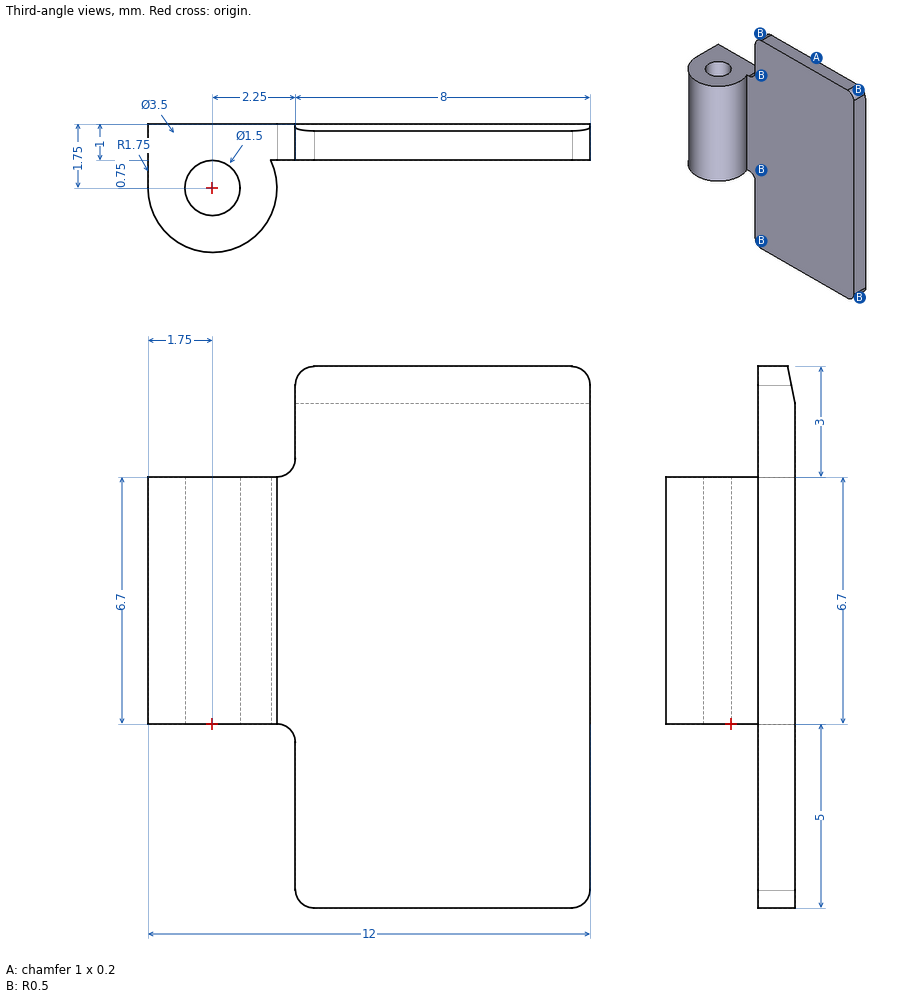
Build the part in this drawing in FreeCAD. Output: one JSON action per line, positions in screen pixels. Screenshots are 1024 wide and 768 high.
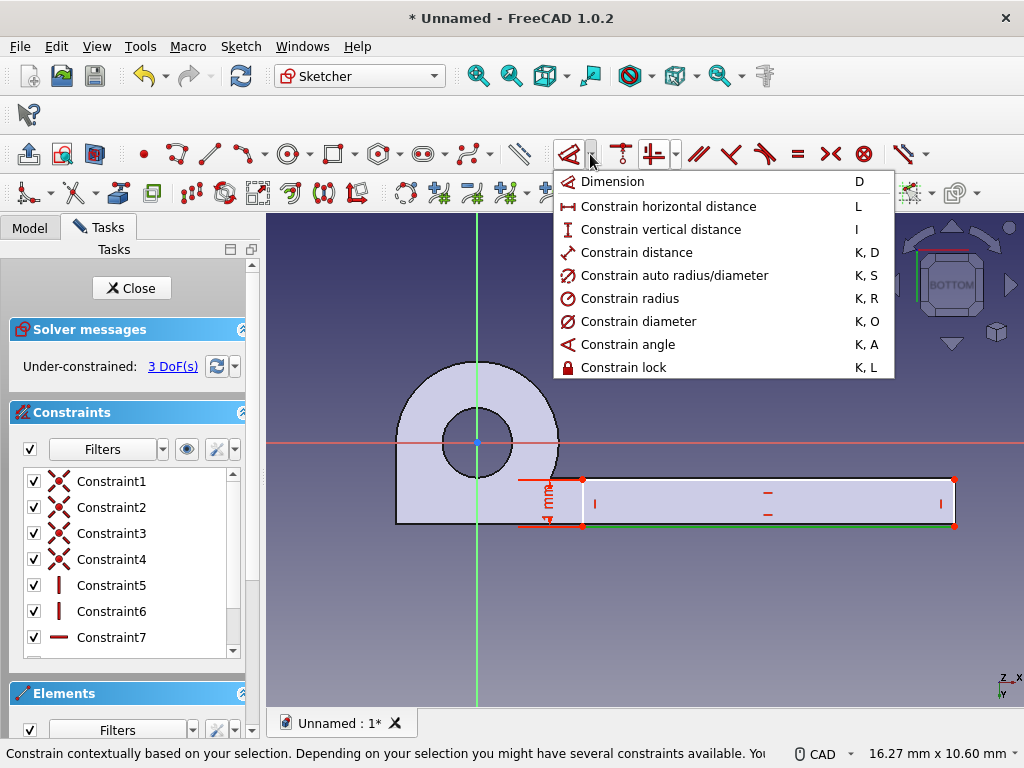
{"action": "left_click", "coordinate": [724, 206]}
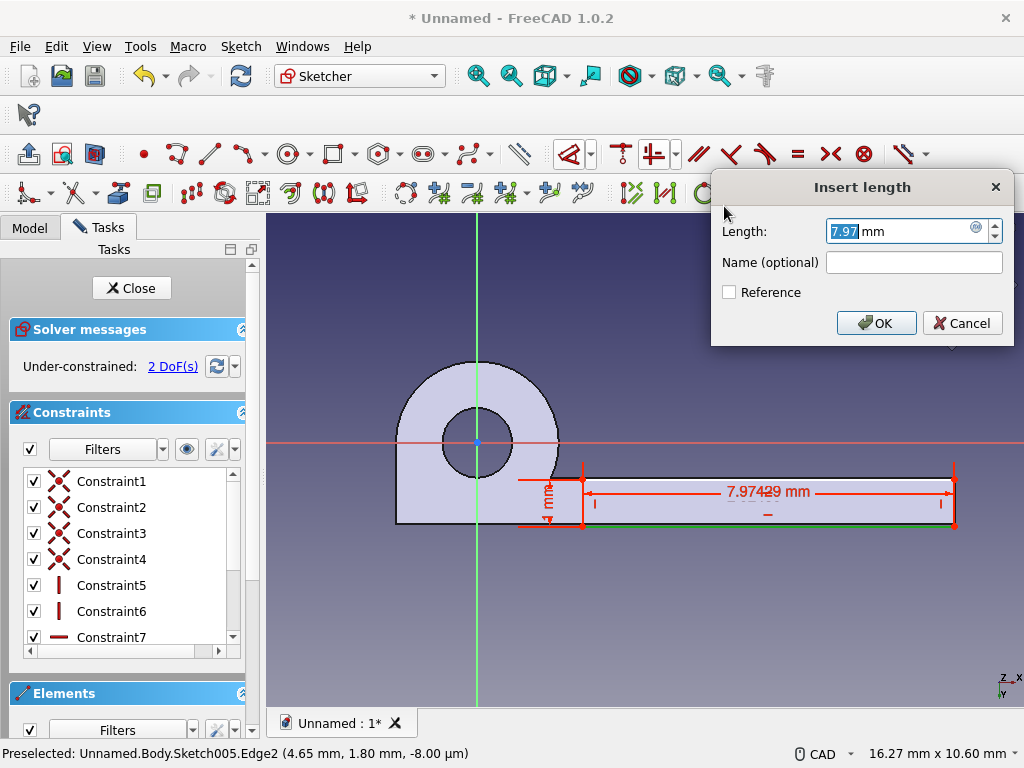
{"action": "type", "text": "8"}
{"action": "key", "text": "Return"}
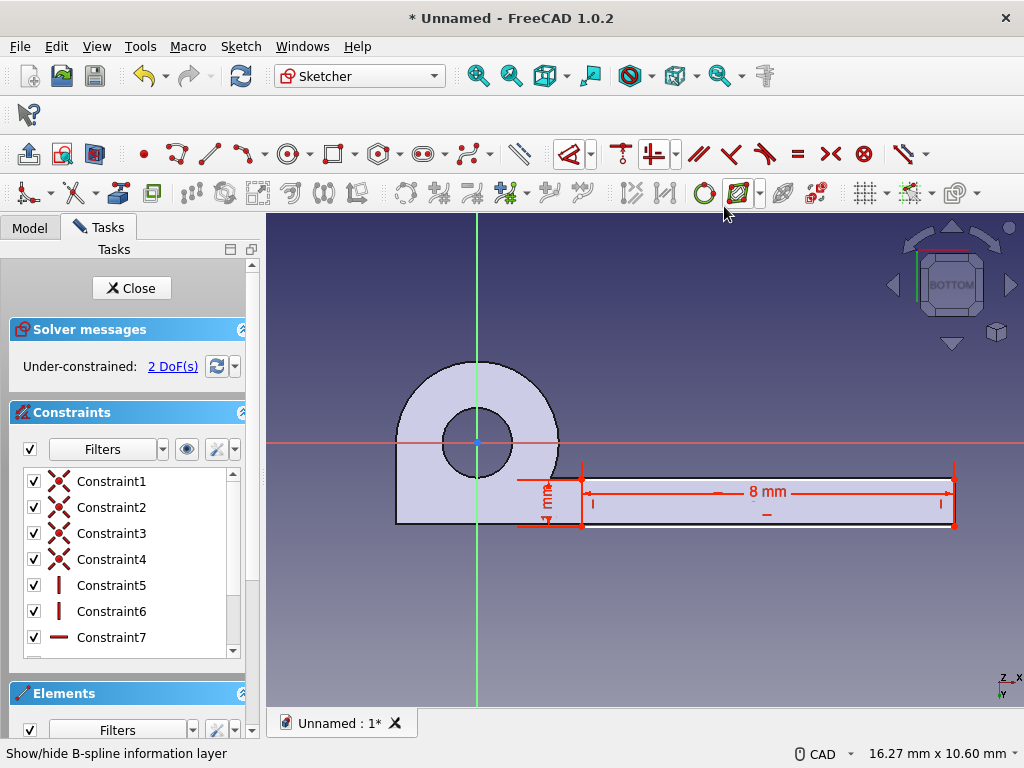
{"action": "left_click", "coordinate": [582, 480]}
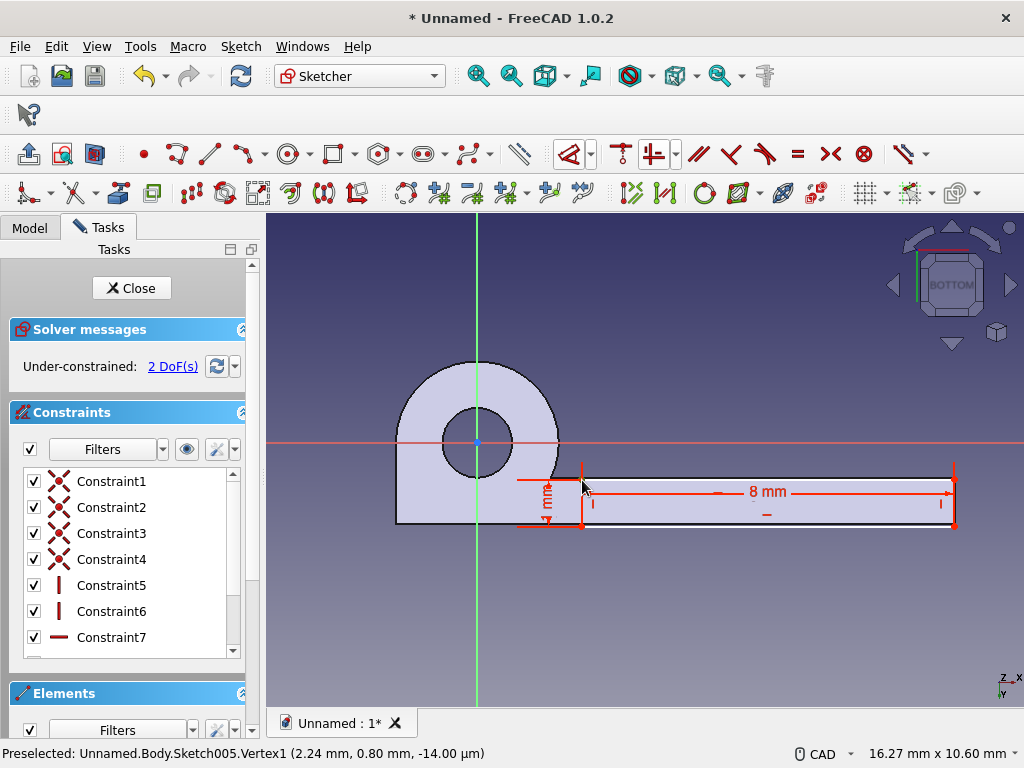
{"action": "key", "text": "l"}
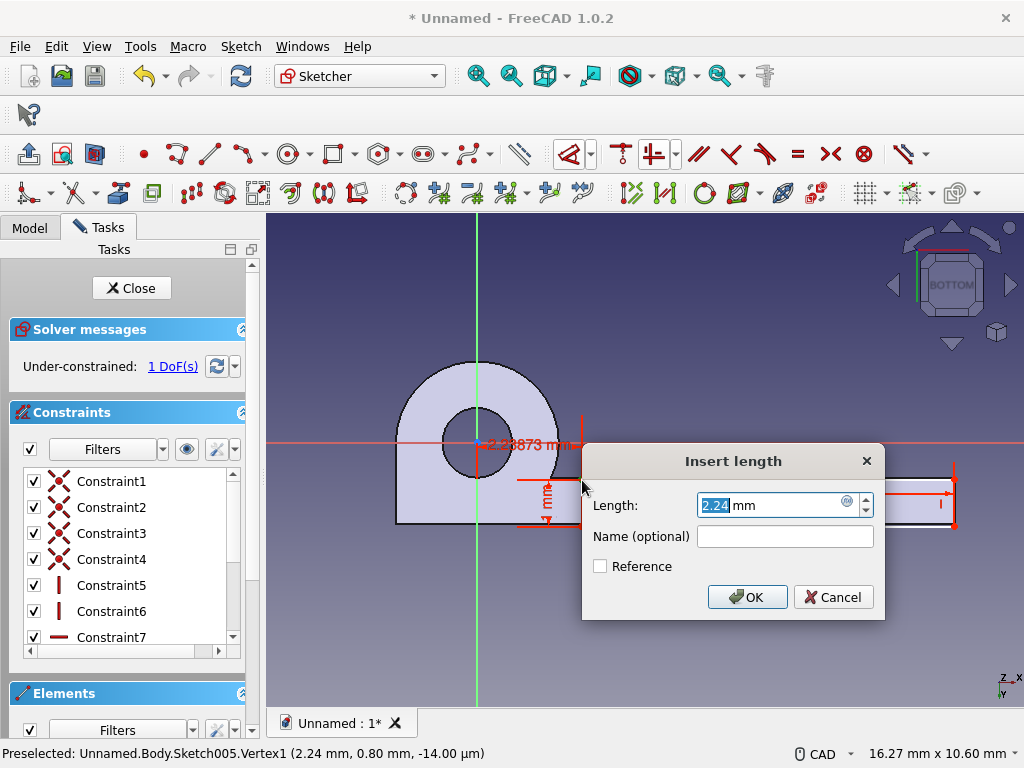
{"action": "type", "text": "2.25"}
{"action": "key", "text": "Return"}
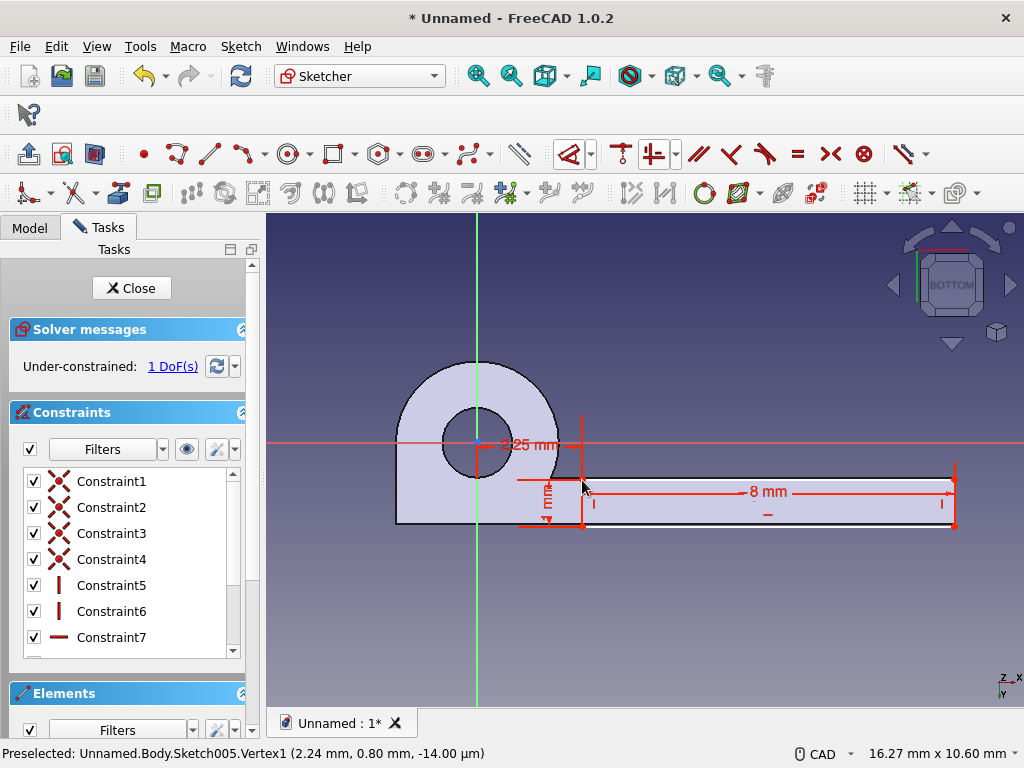
{"action": "left_click", "coordinate": [582, 480]}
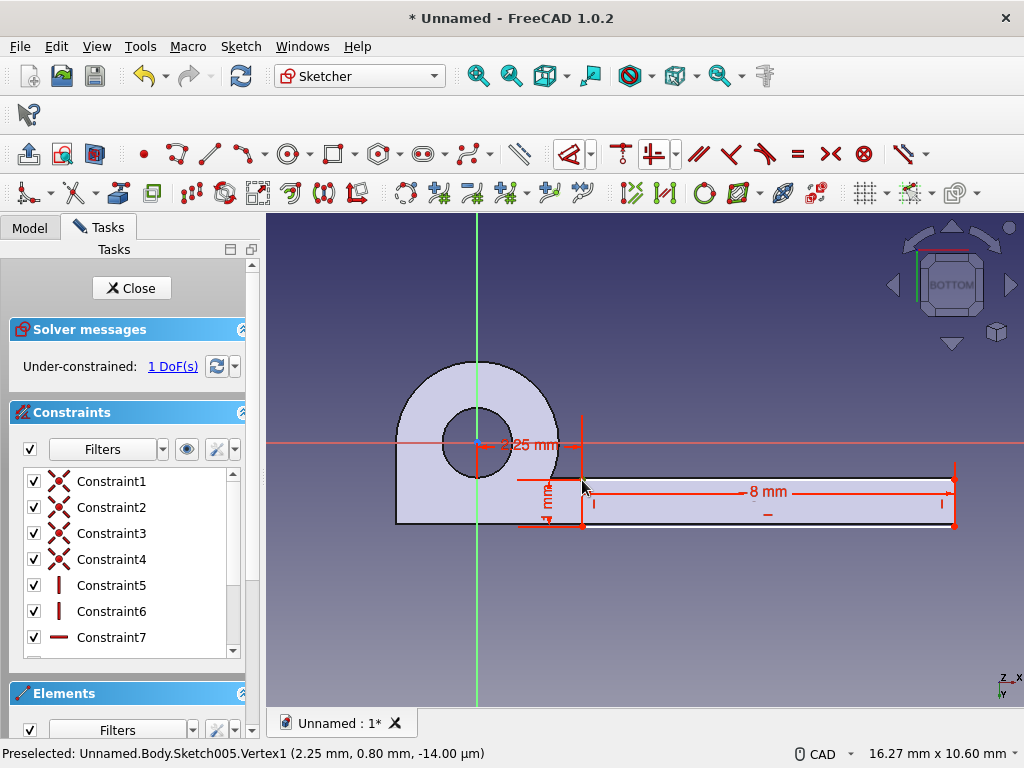
{"action": "left_click", "coordinate": [590, 154]}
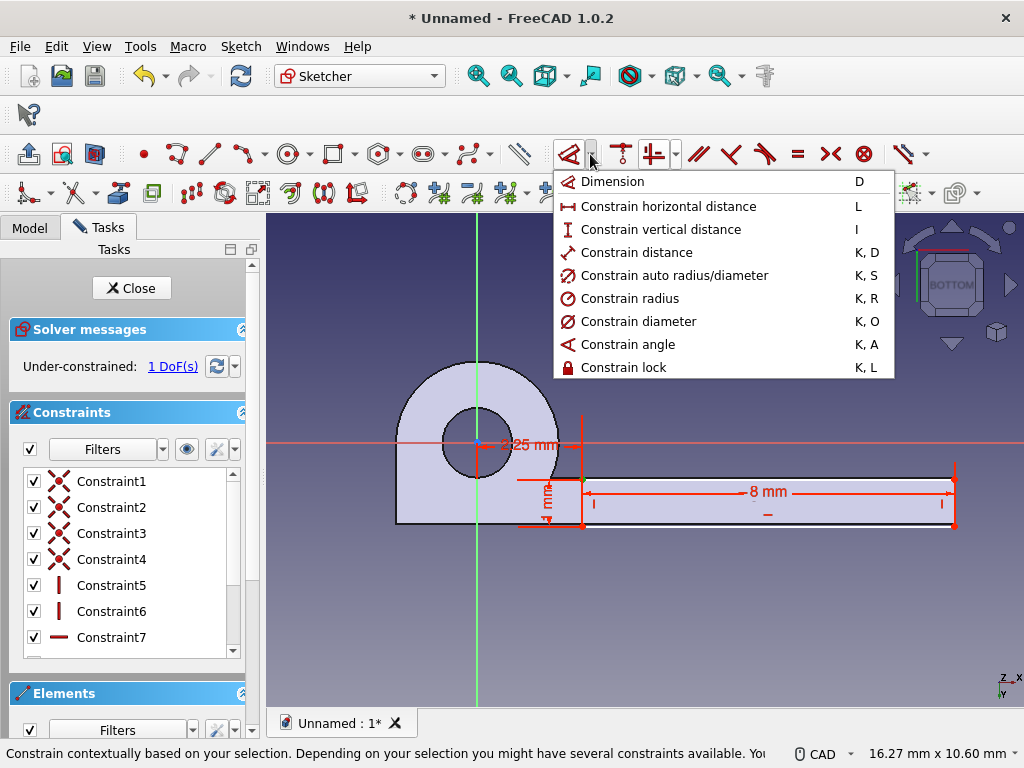
{"action": "left_click", "coordinate": [724, 230]}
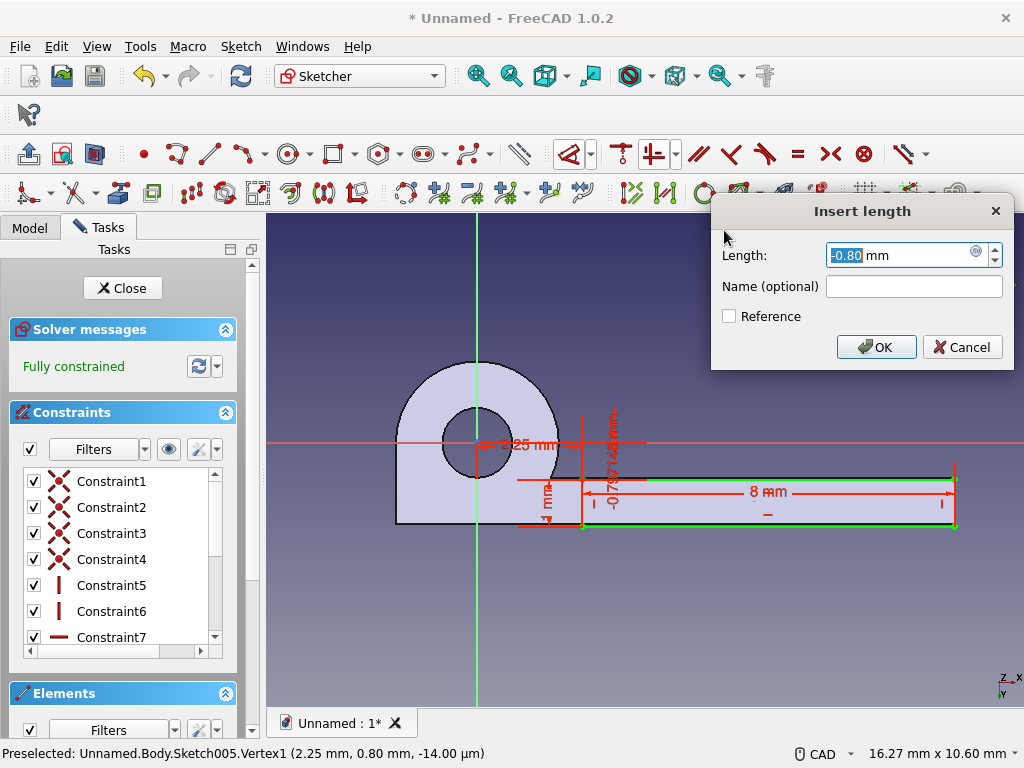
{"action": "type", "text": "-0.75"}
{"action": "key", "text": "Return"}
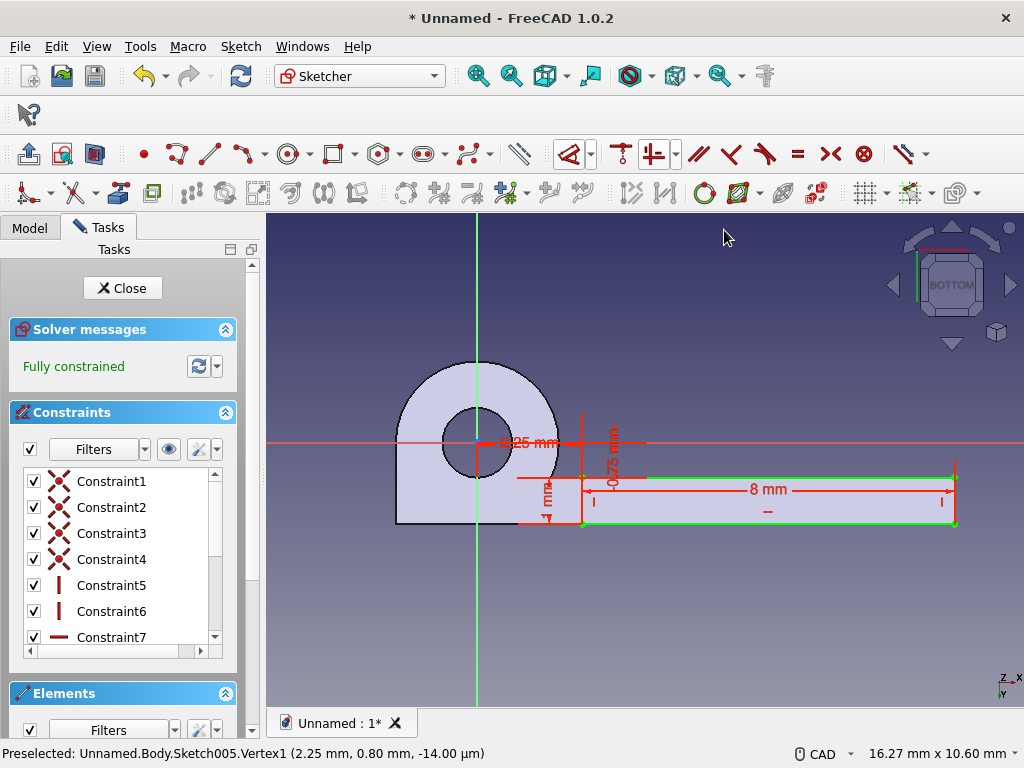
{"action": "left_click", "coordinate": [123, 288]}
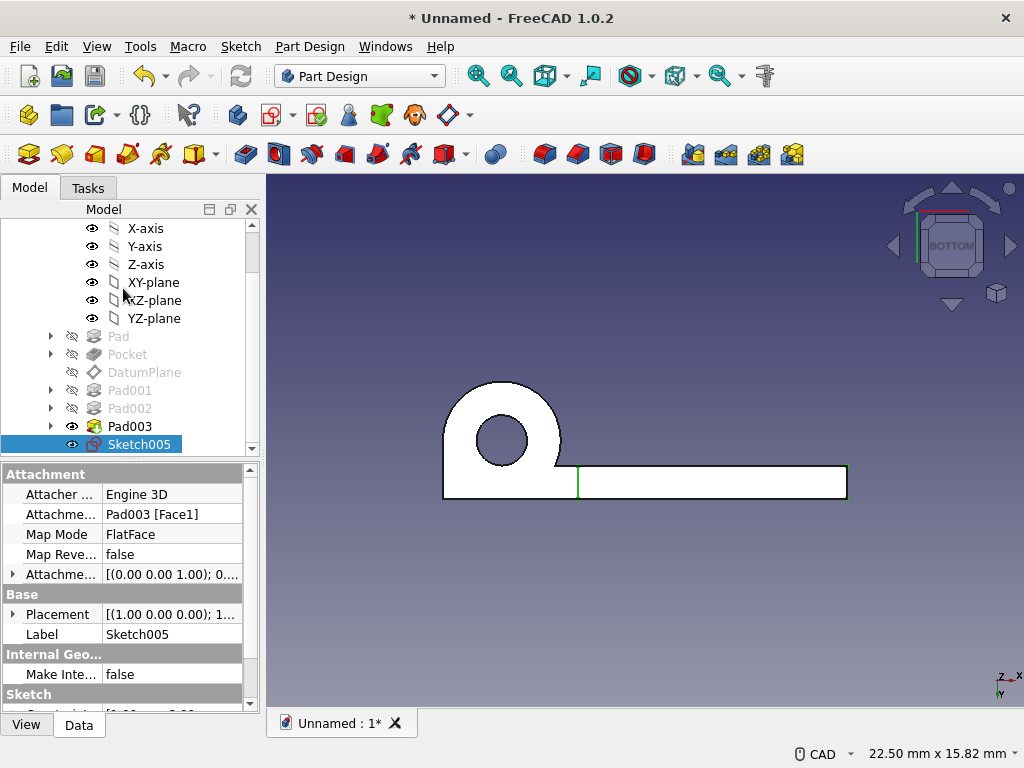
{"action": "left_click", "coordinate": [29, 154]}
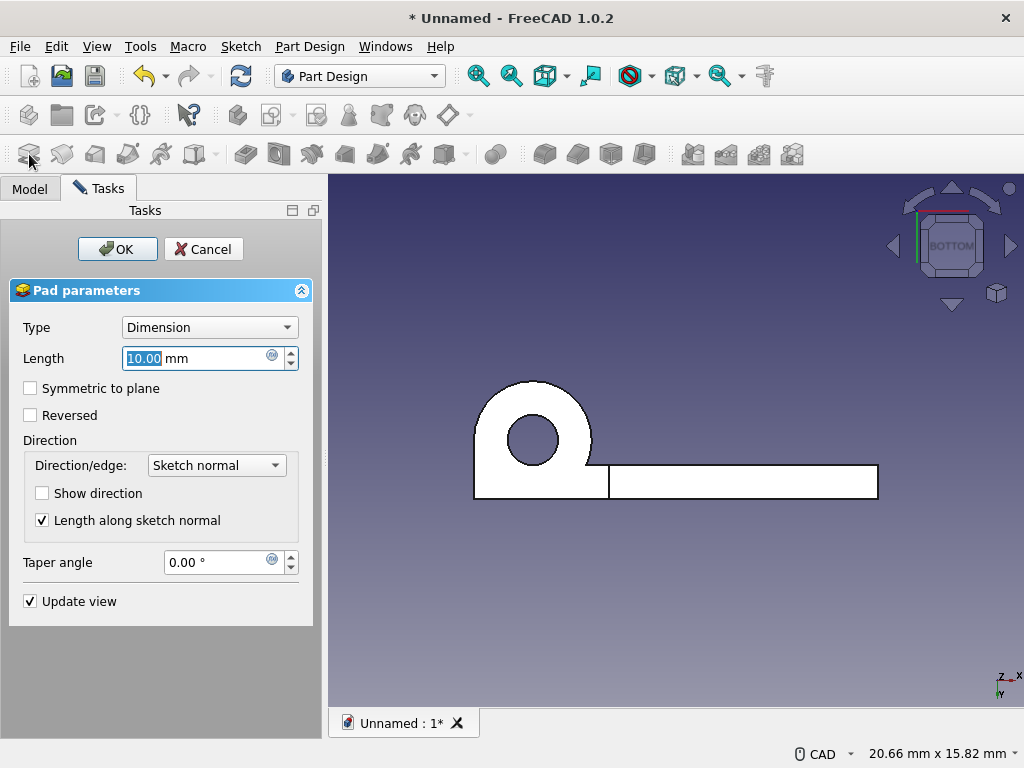
{"action": "type", "text": "5"}
{"action": "key", "text": "Tab"}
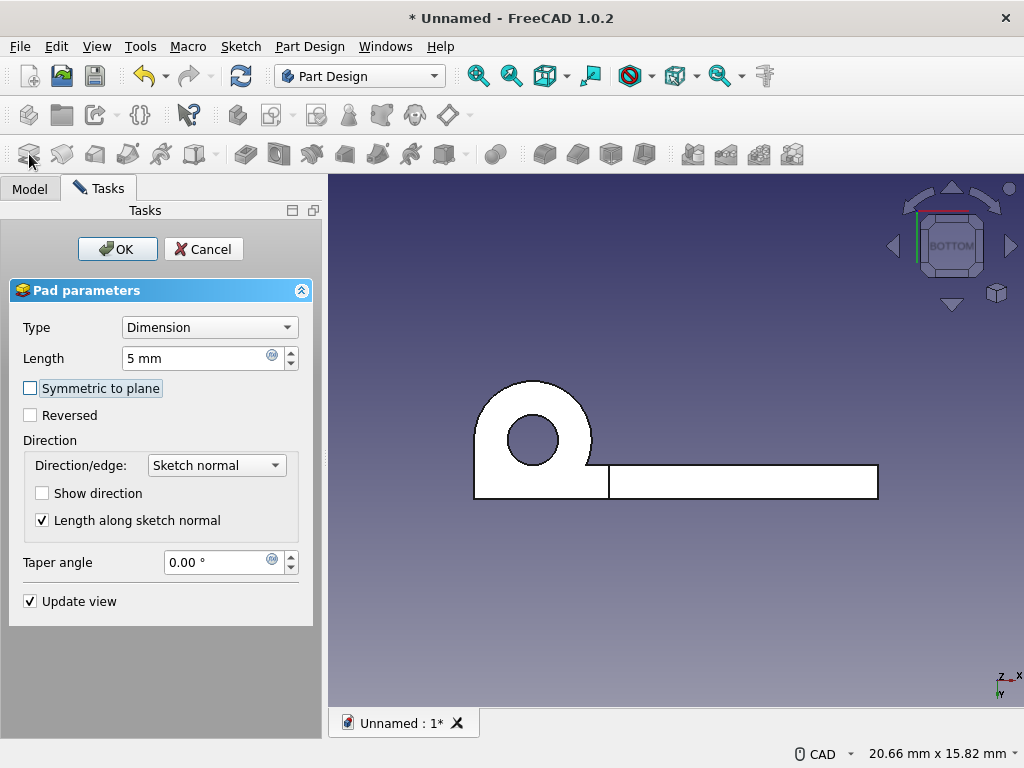
{"action": "left_click", "coordinate": [118, 249]}